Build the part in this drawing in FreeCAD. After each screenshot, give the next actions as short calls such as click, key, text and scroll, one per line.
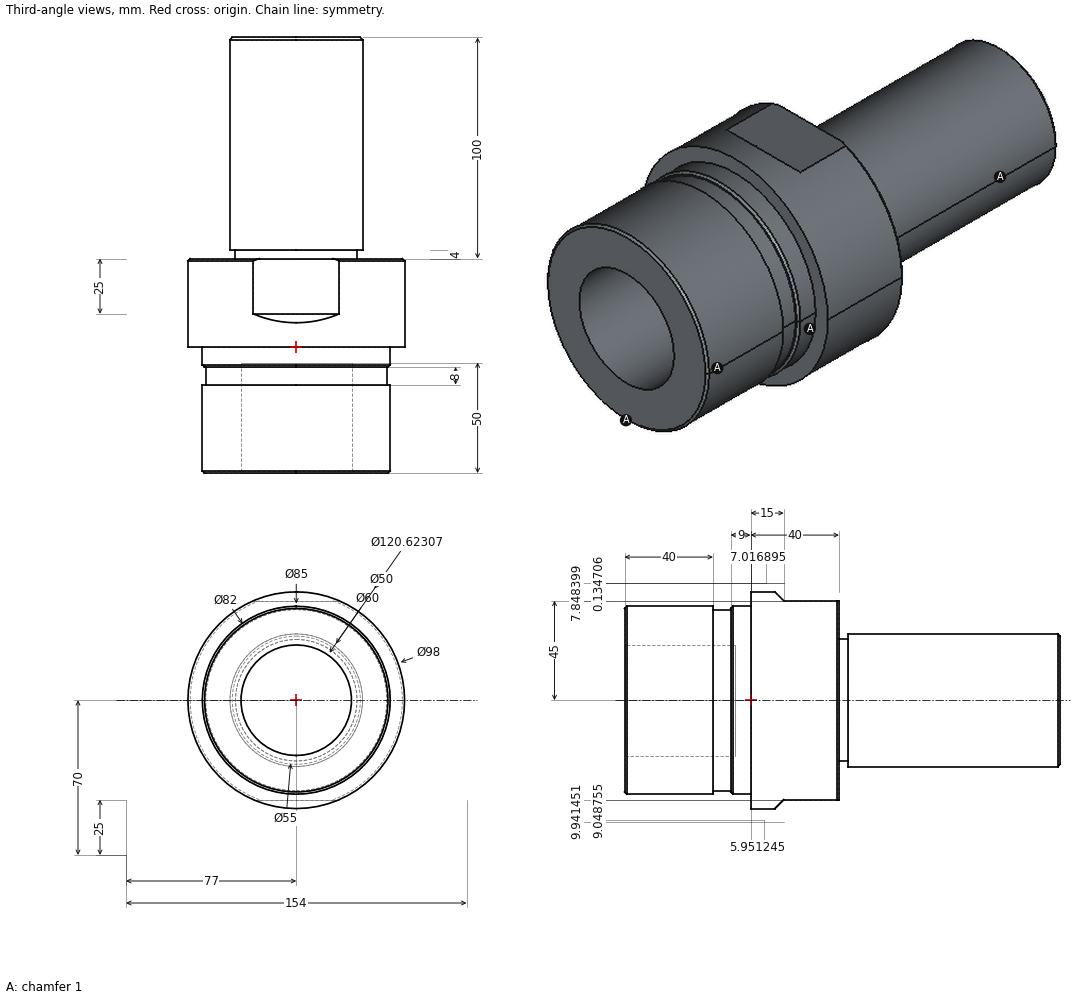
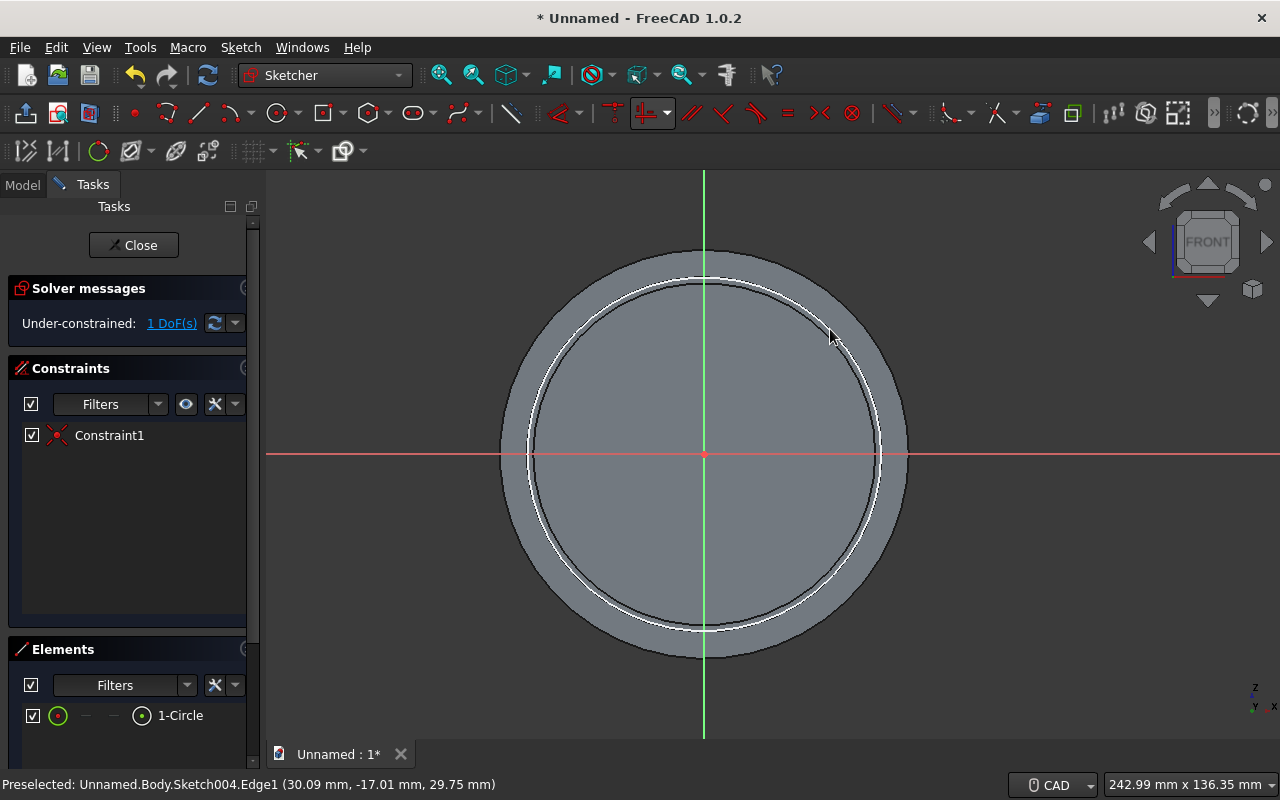
click(558, 114)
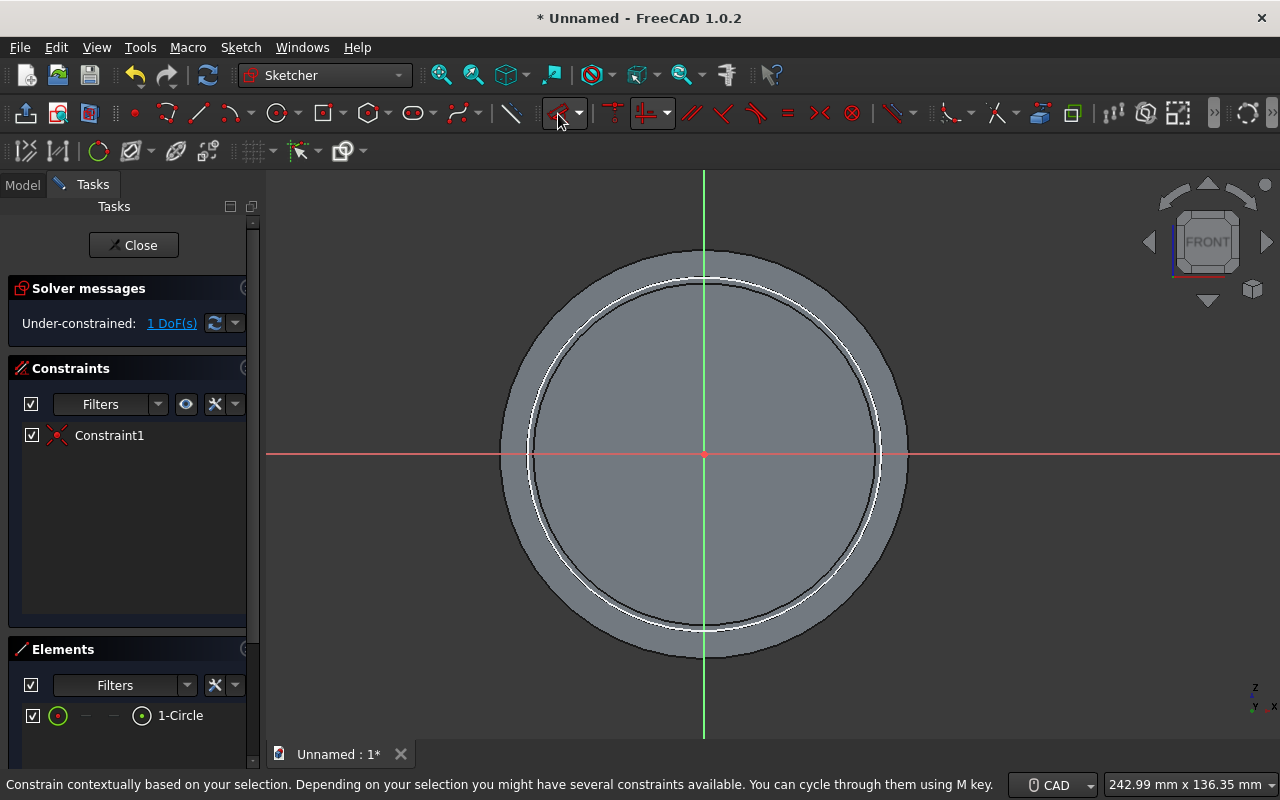
click(829, 329)
click(852, 306)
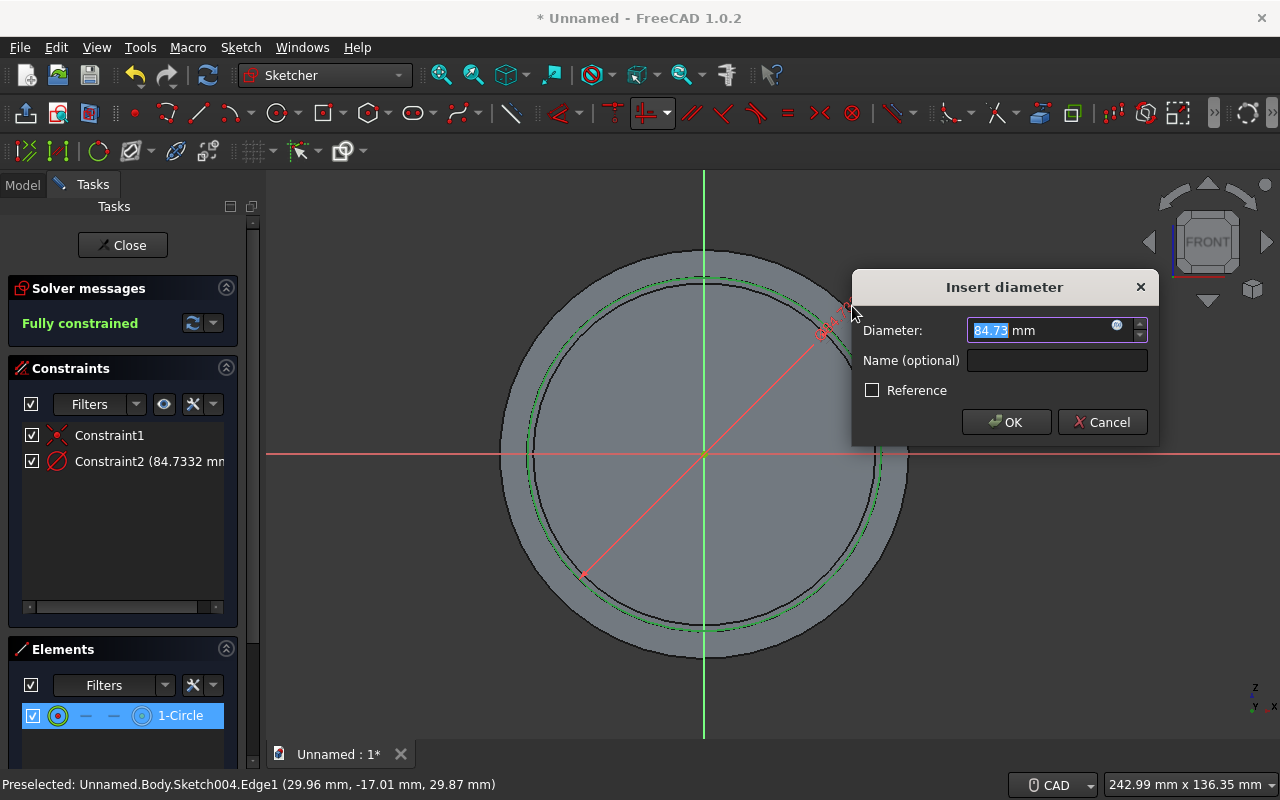
text(85)
key(Return)
key(Escape)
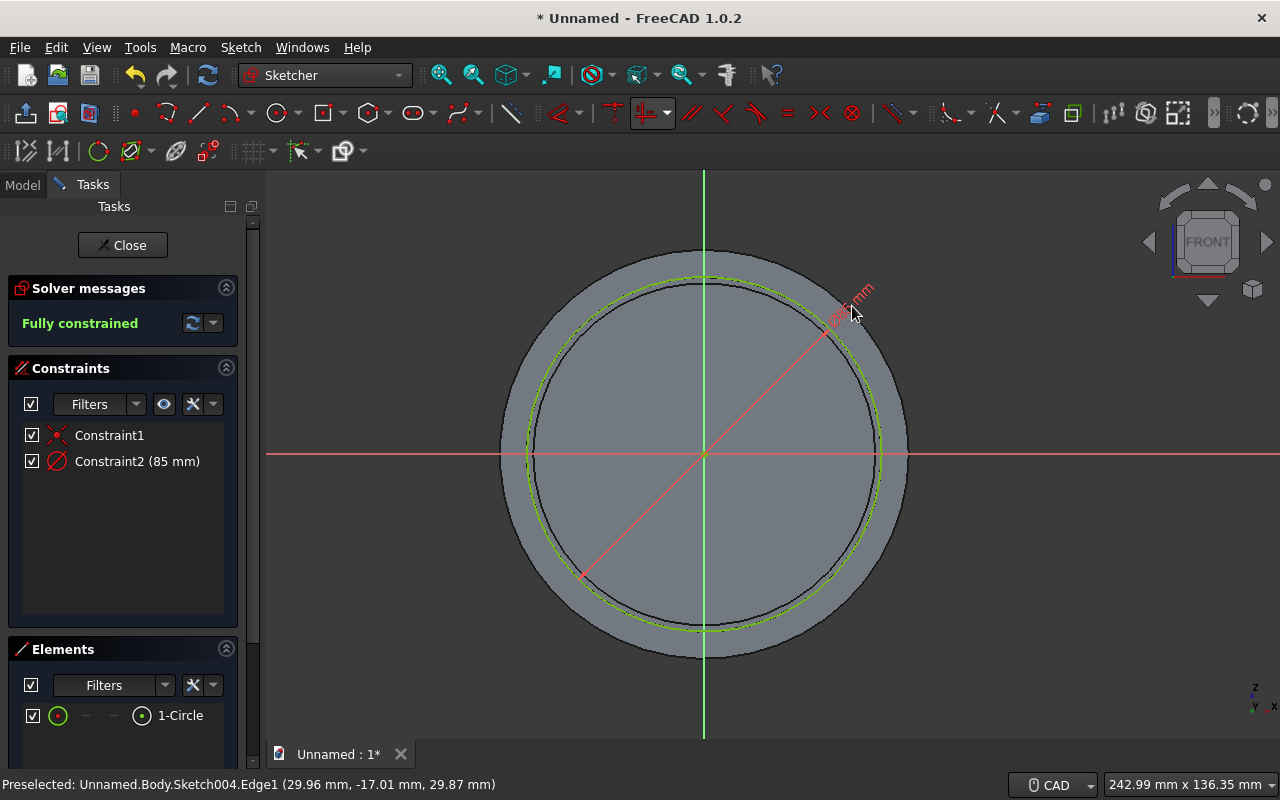
click(123, 245)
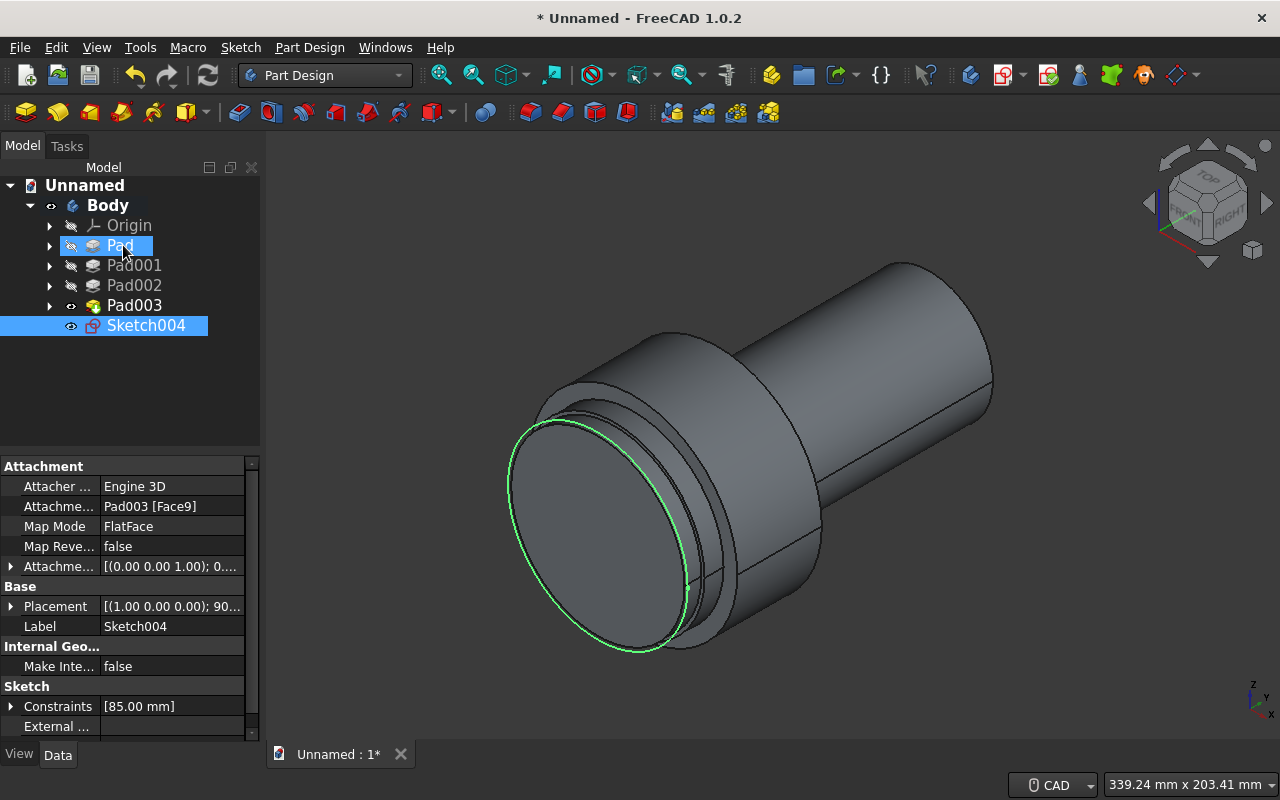
click(26, 112)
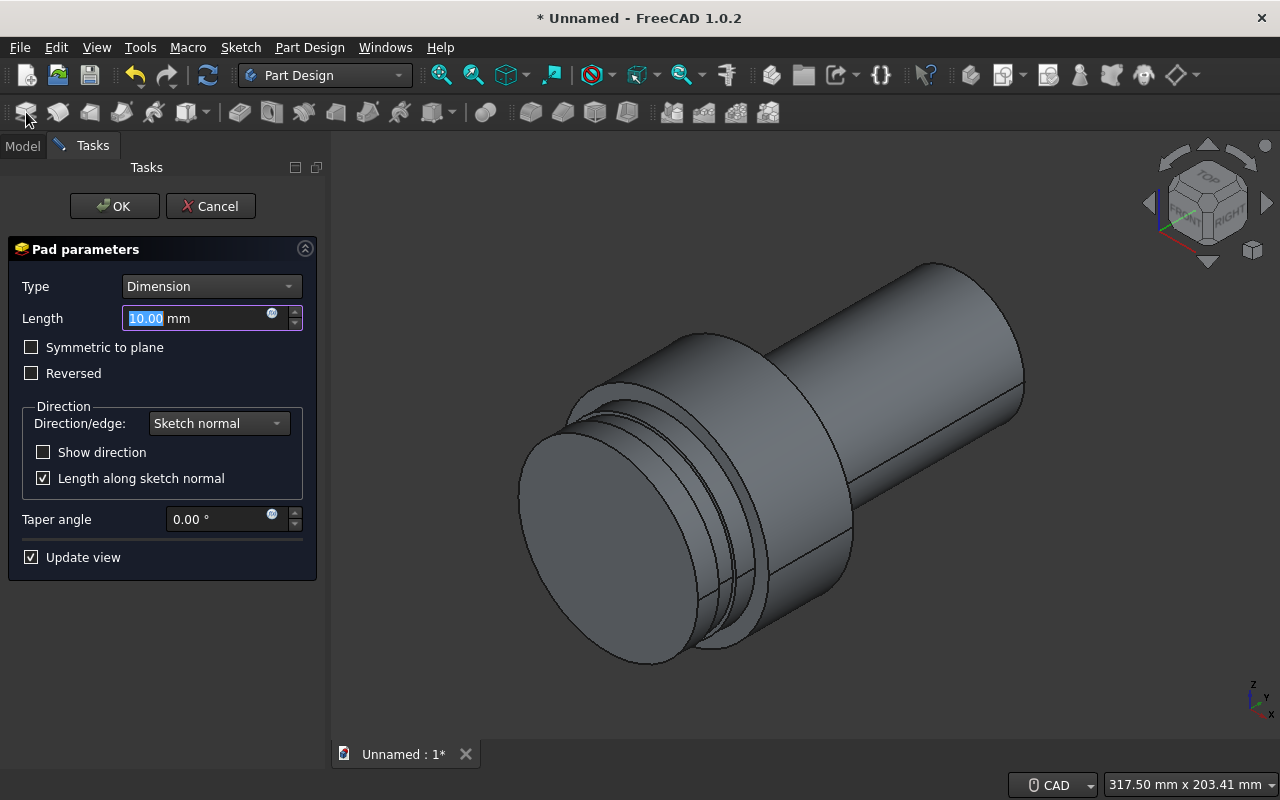
text(40)
key(Tab)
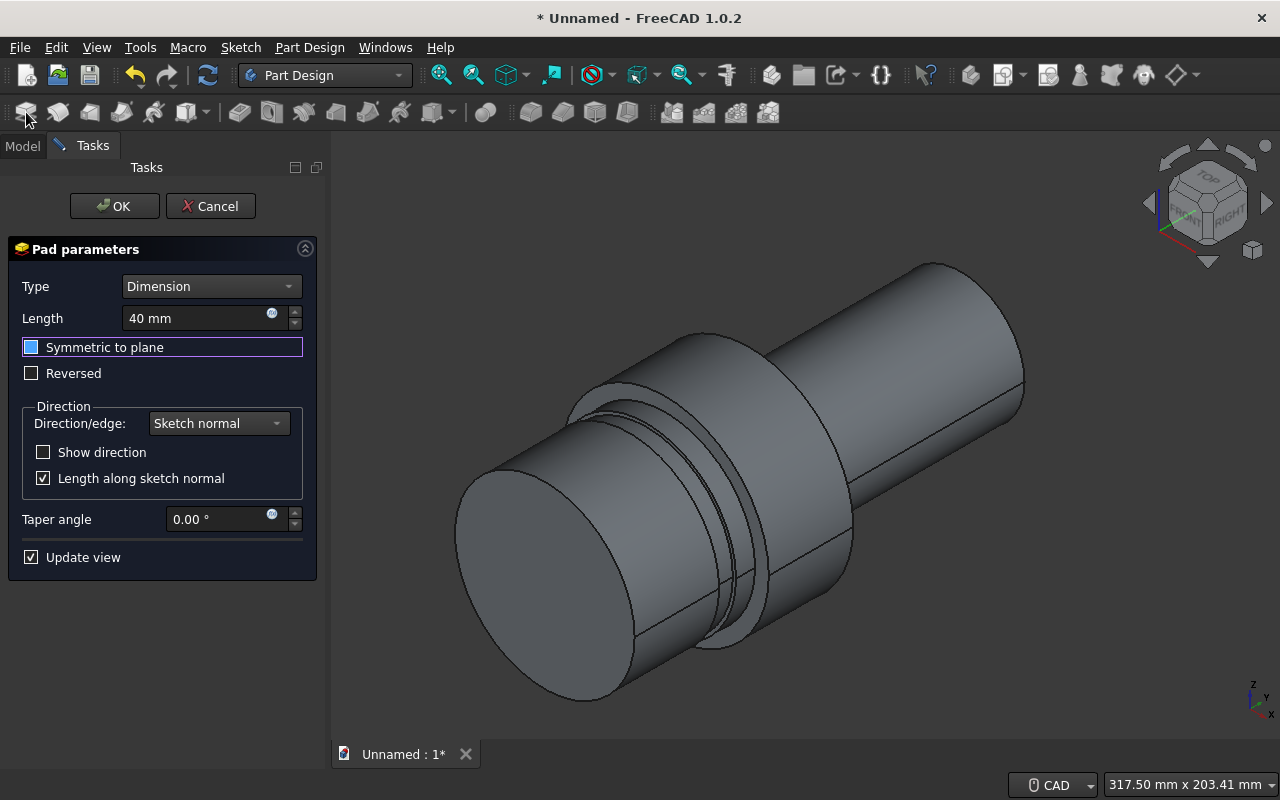
click(115, 206)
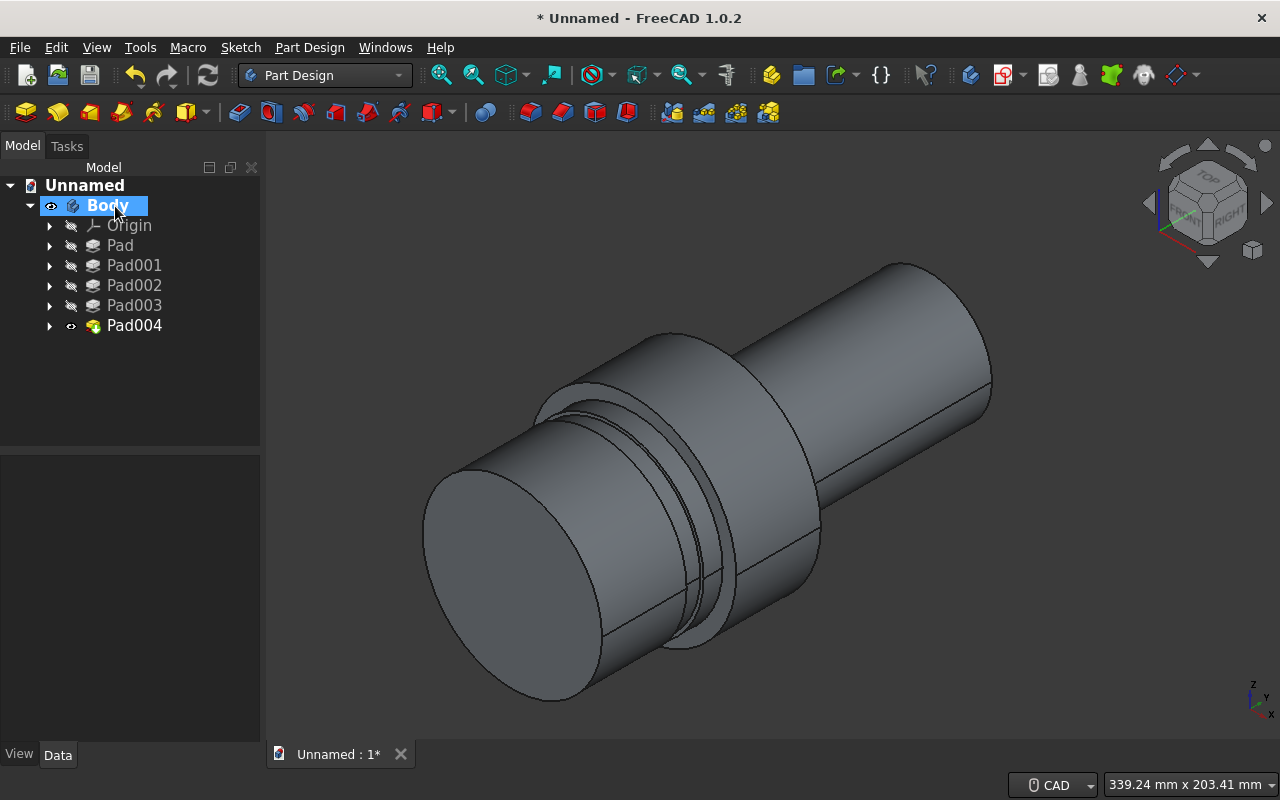
click(442, 76)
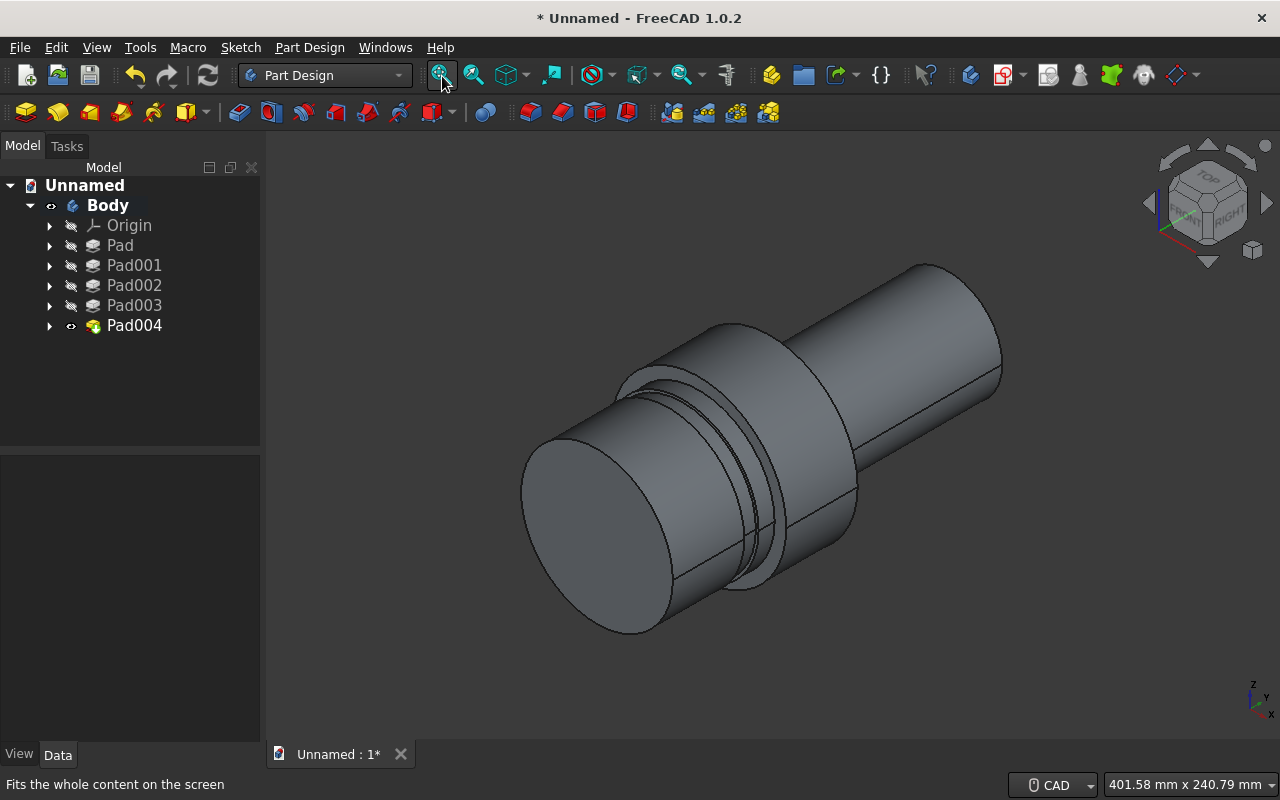
click(706, 416)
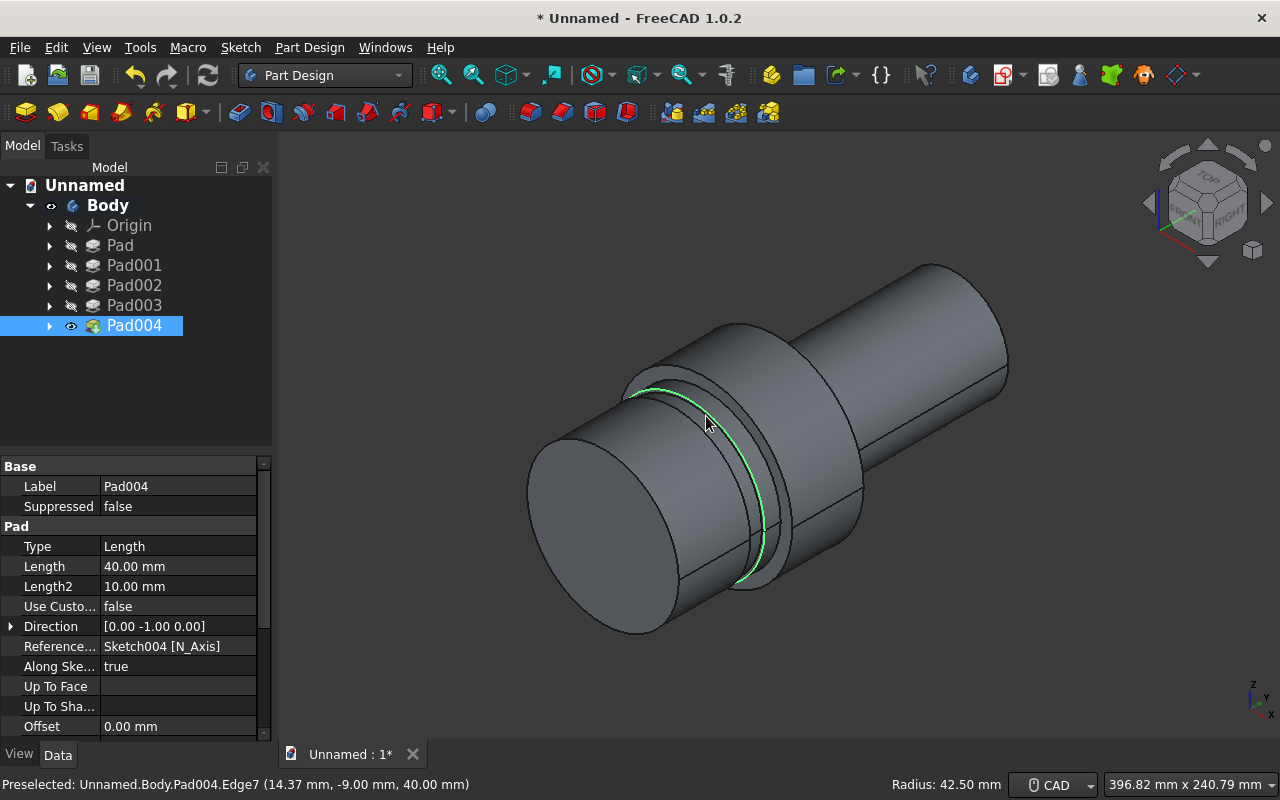
click(580, 439, ctrl)